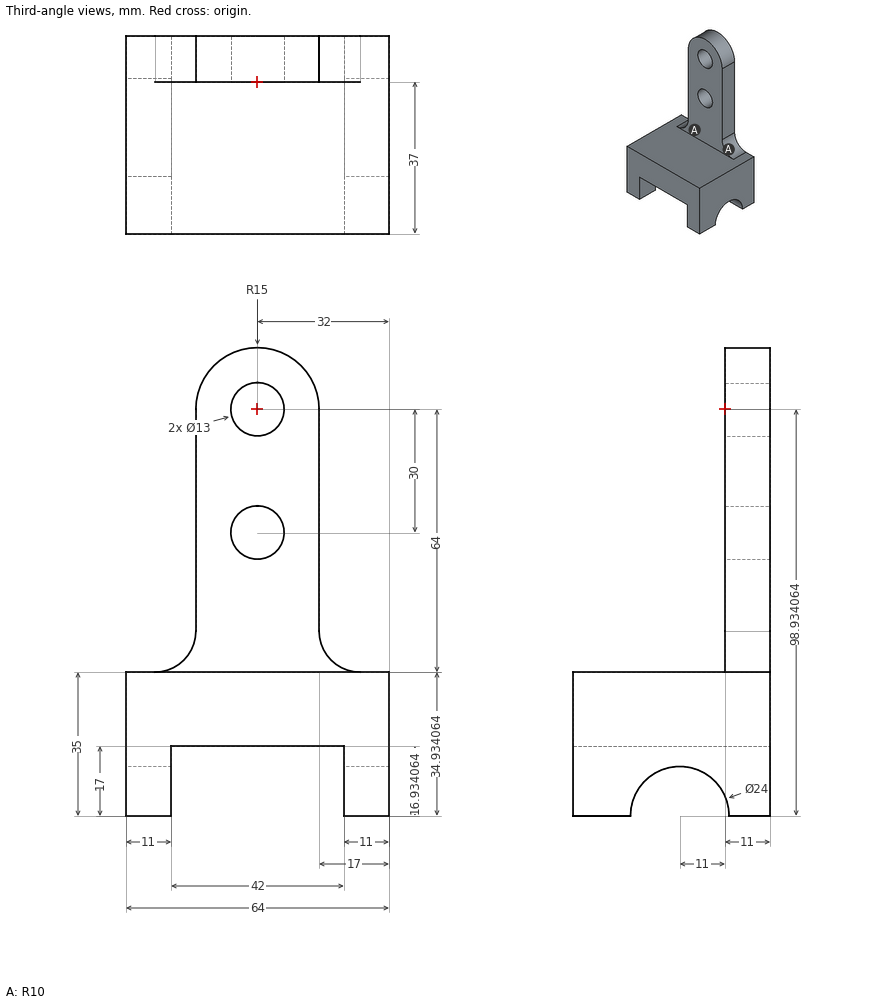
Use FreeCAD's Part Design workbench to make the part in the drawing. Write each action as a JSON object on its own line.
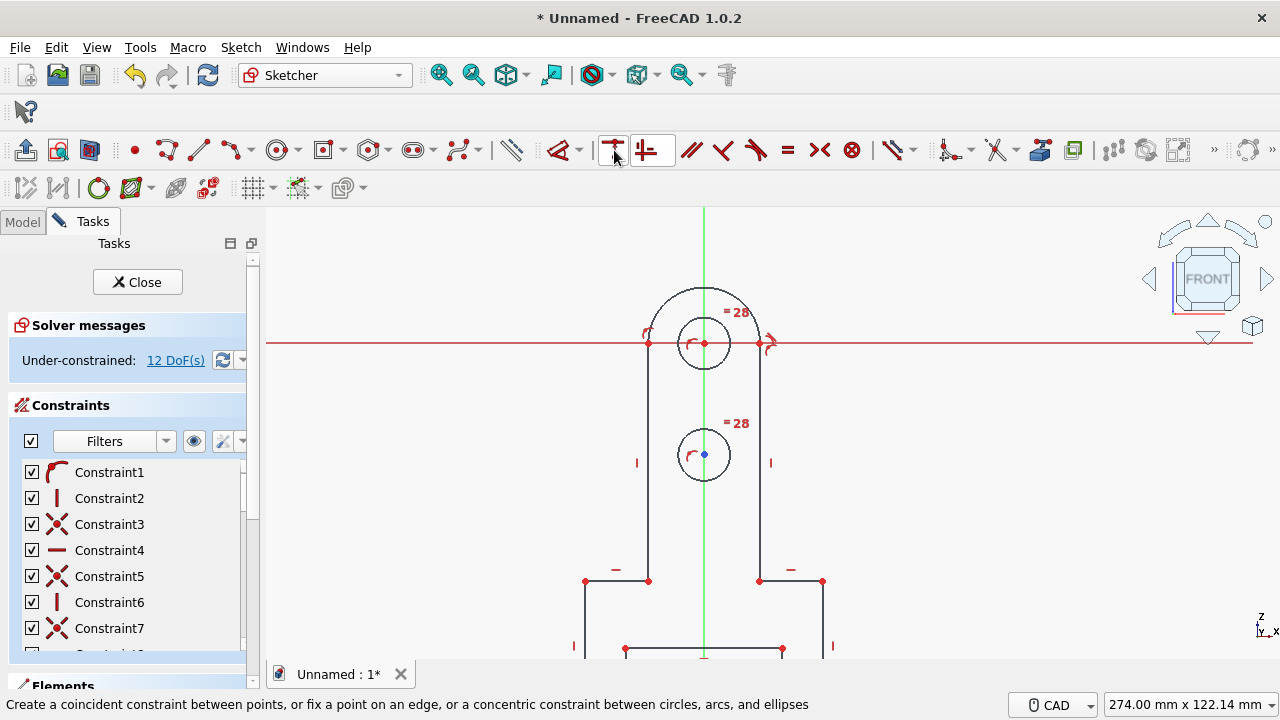
{"action": "left_click", "coordinate": [737, 298]}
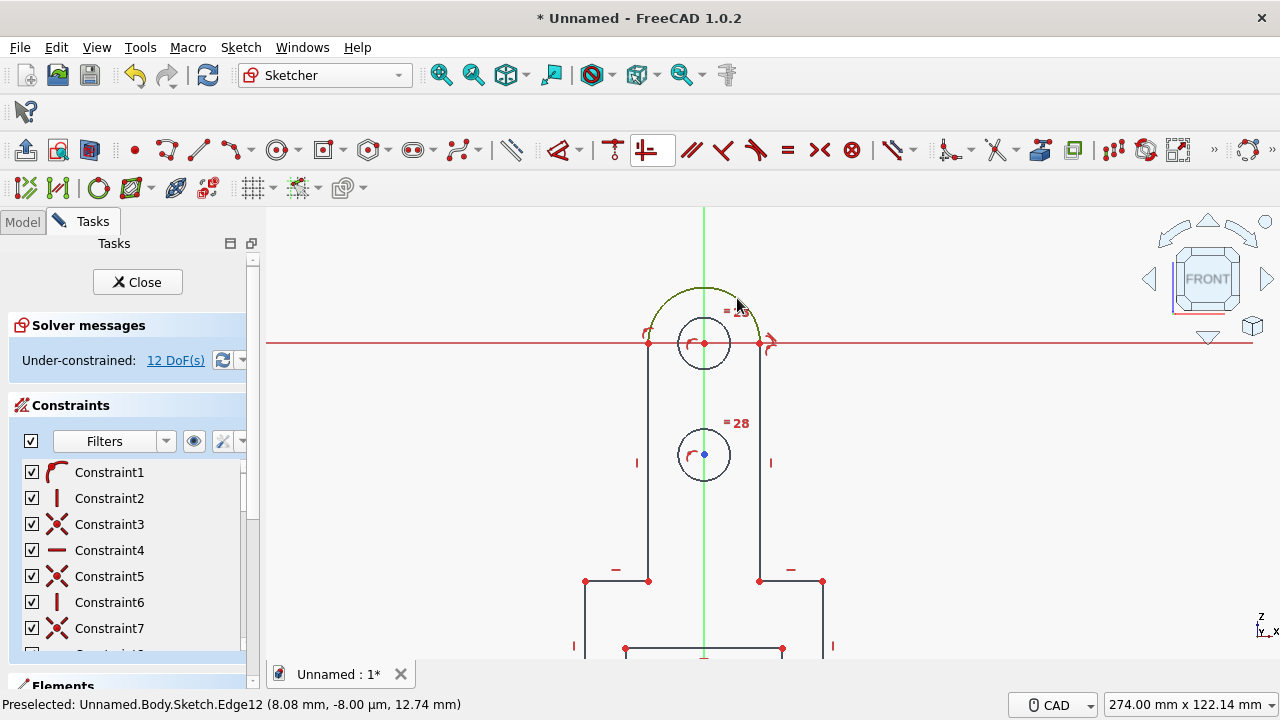
{"action": "left_click", "coordinate": [582, 150]}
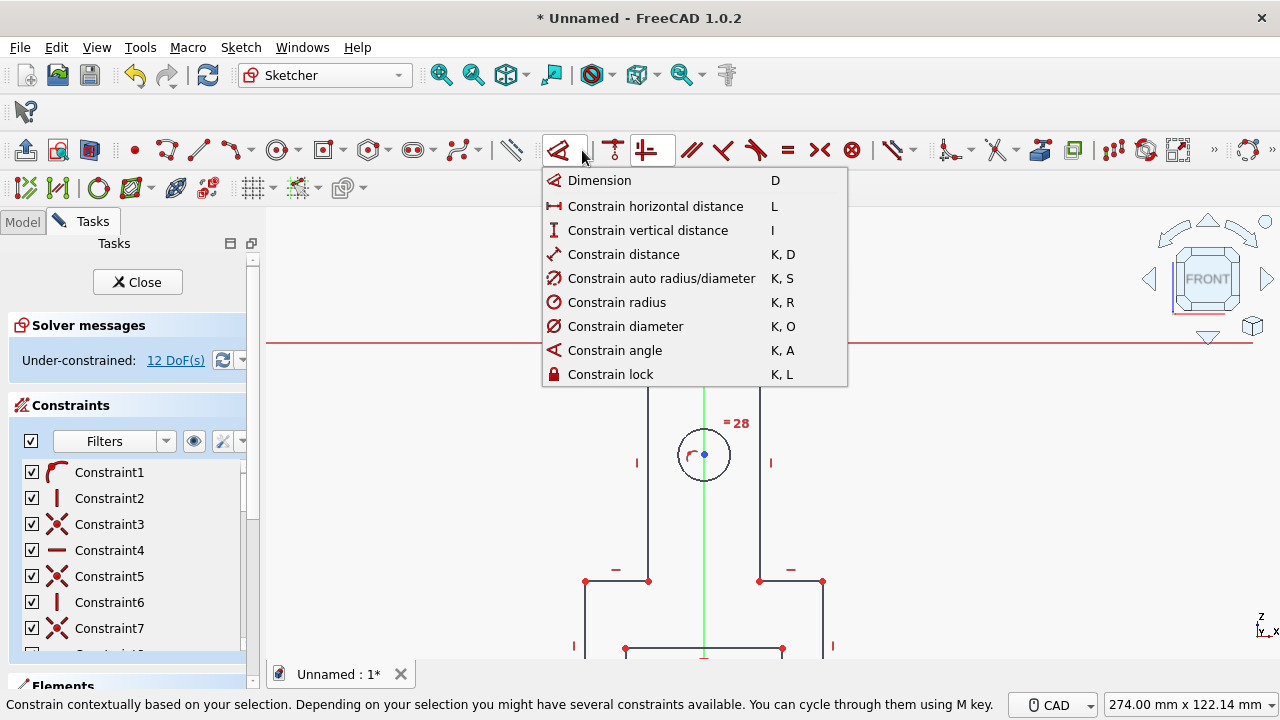
{"action": "left_click", "coordinate": [695, 302]}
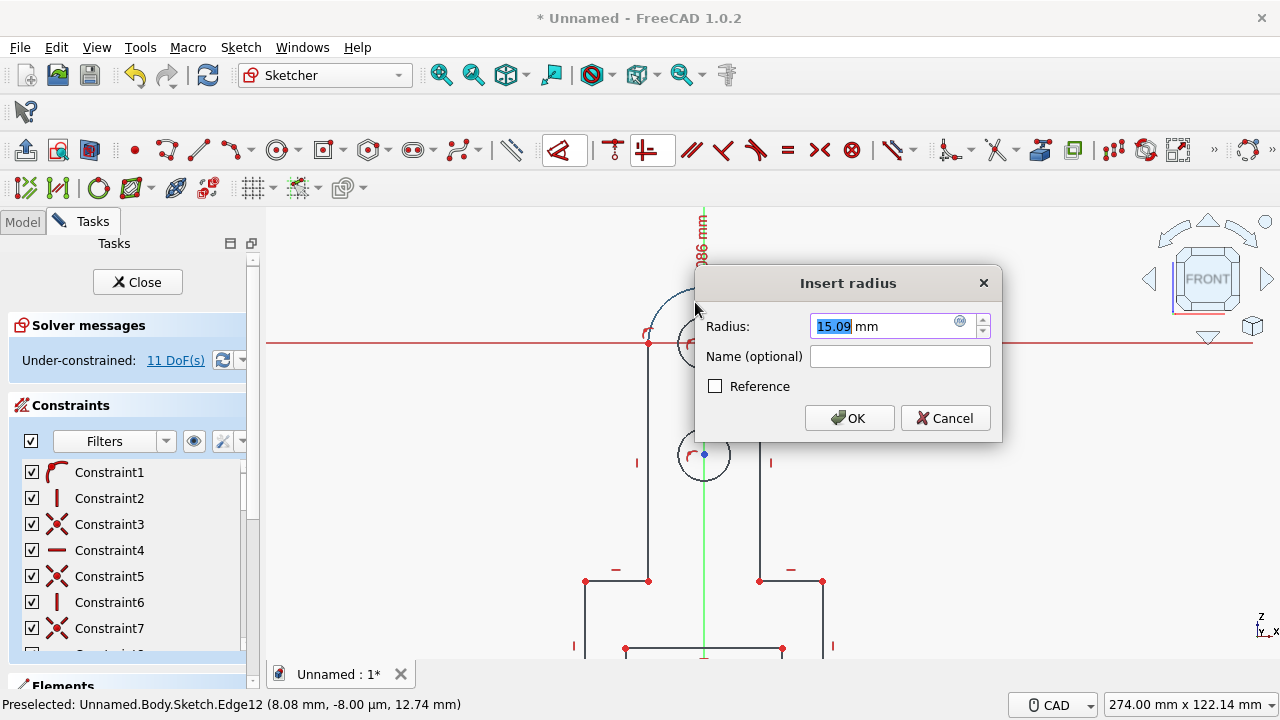
{"action": "type", "text": "15"}
{"action": "key", "text": "Return"}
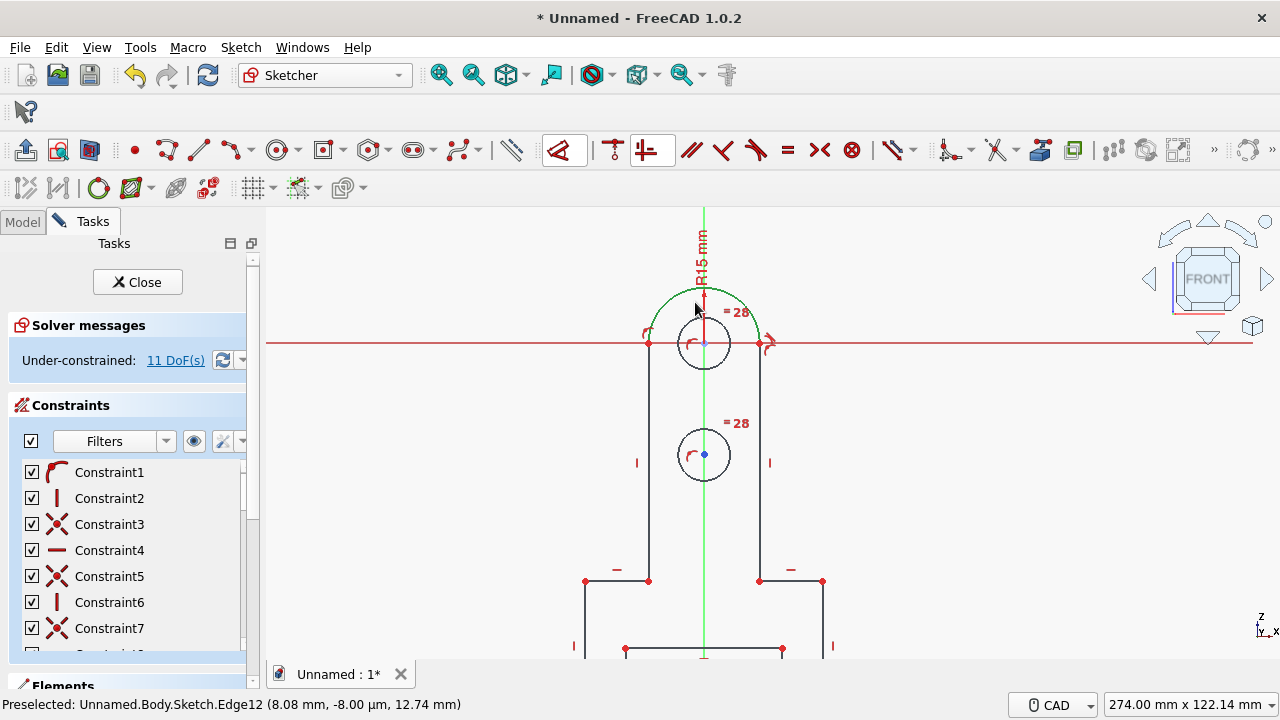
{"action": "left_click", "coordinate": [722, 325]}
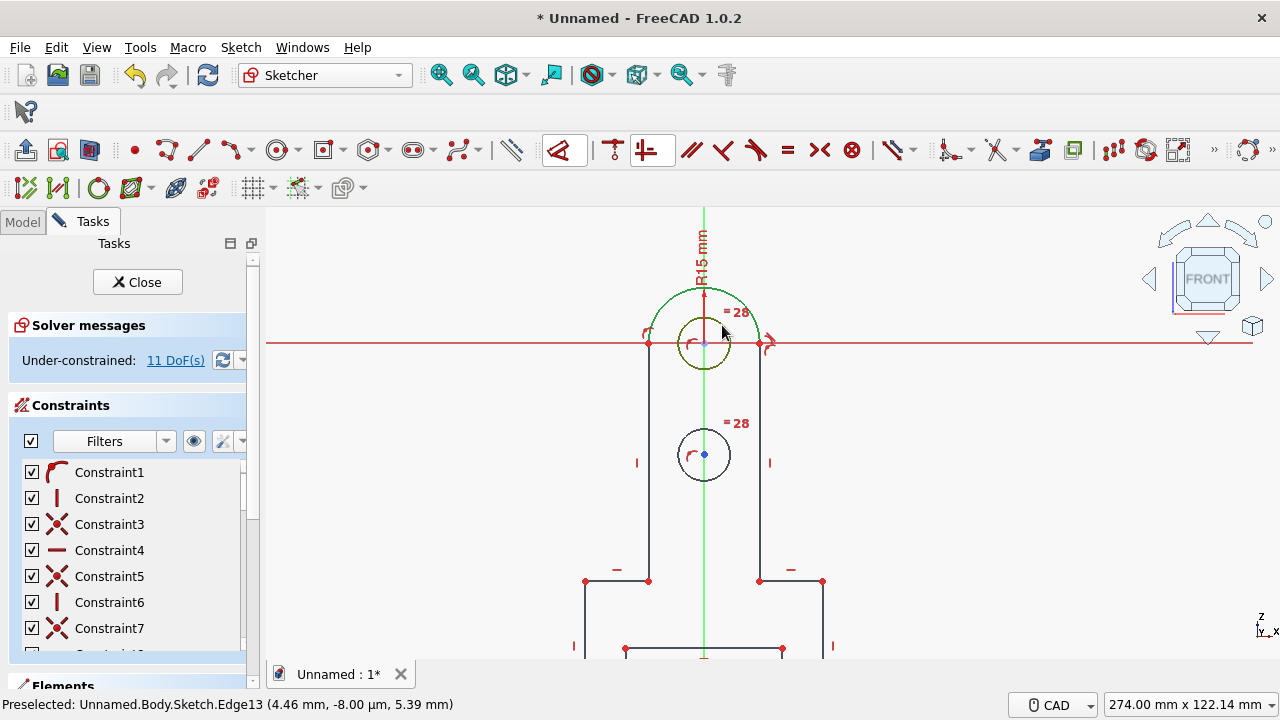
{"action": "left_click", "coordinate": [582, 150]}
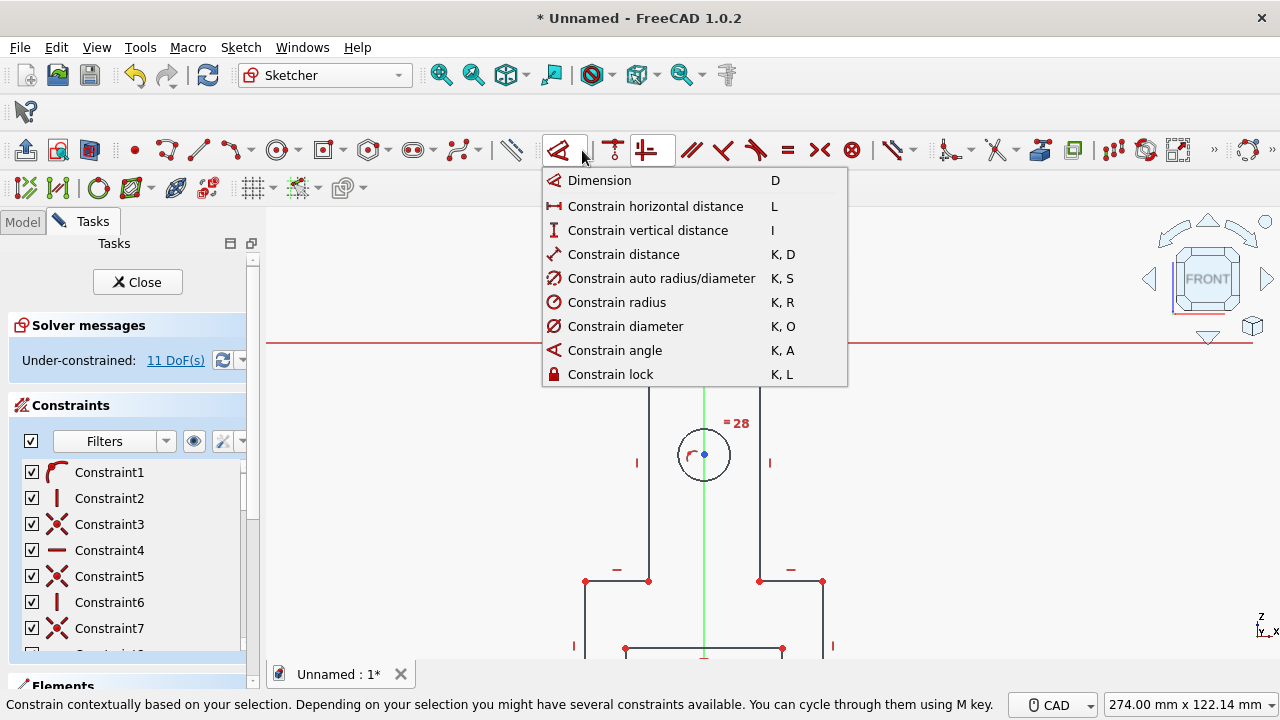
{"action": "left_click", "coordinate": [695, 326]}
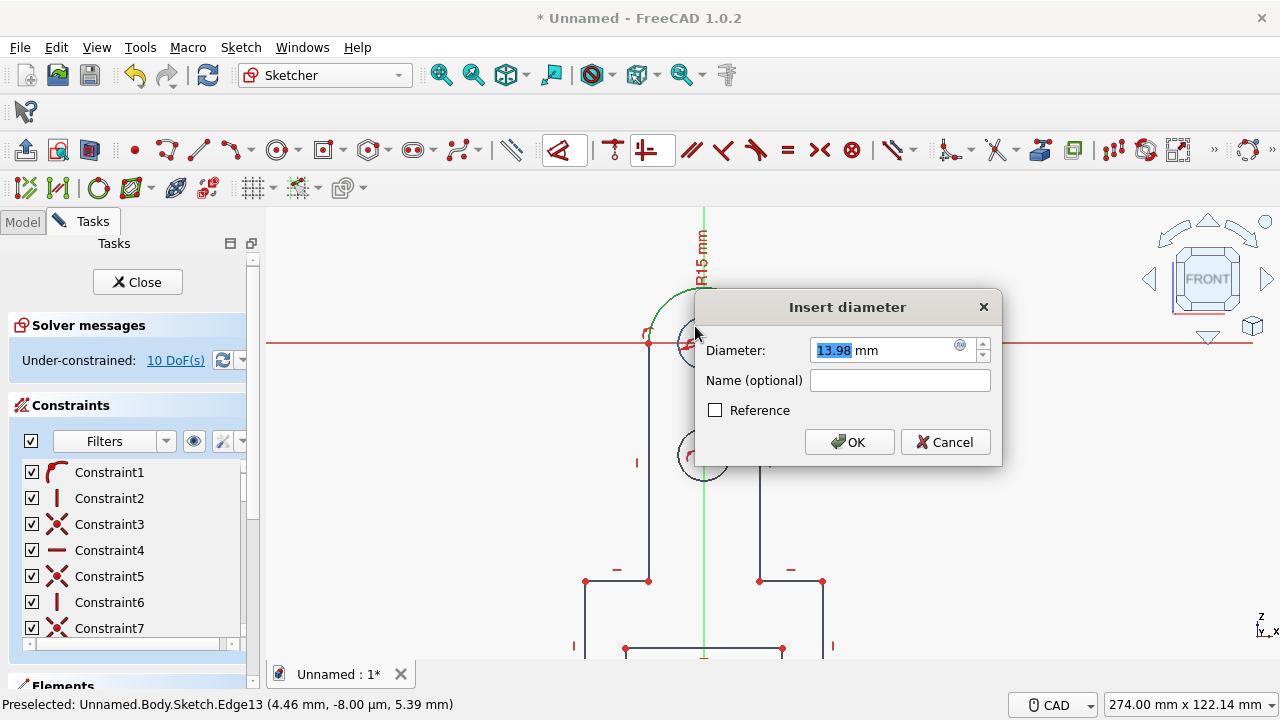
{"action": "type", "text": "13"}
{"action": "key", "text": "Return"}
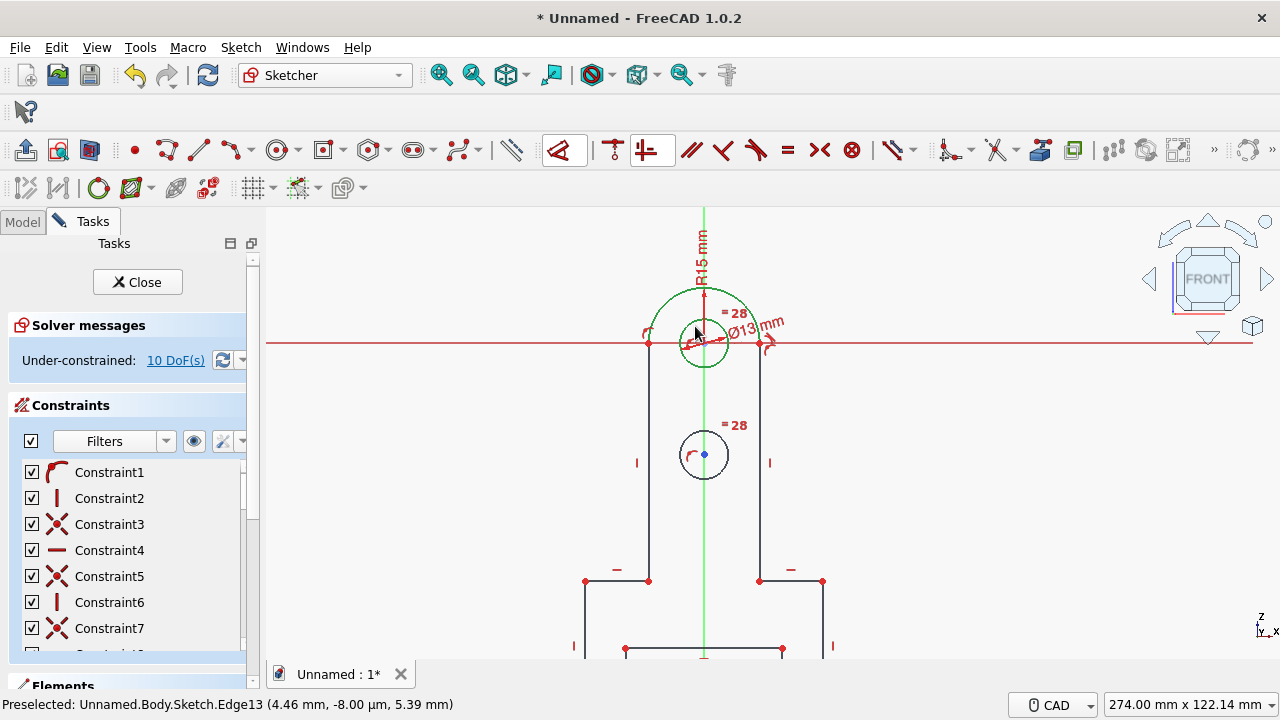
{"action": "left_click", "coordinate": [760, 415]}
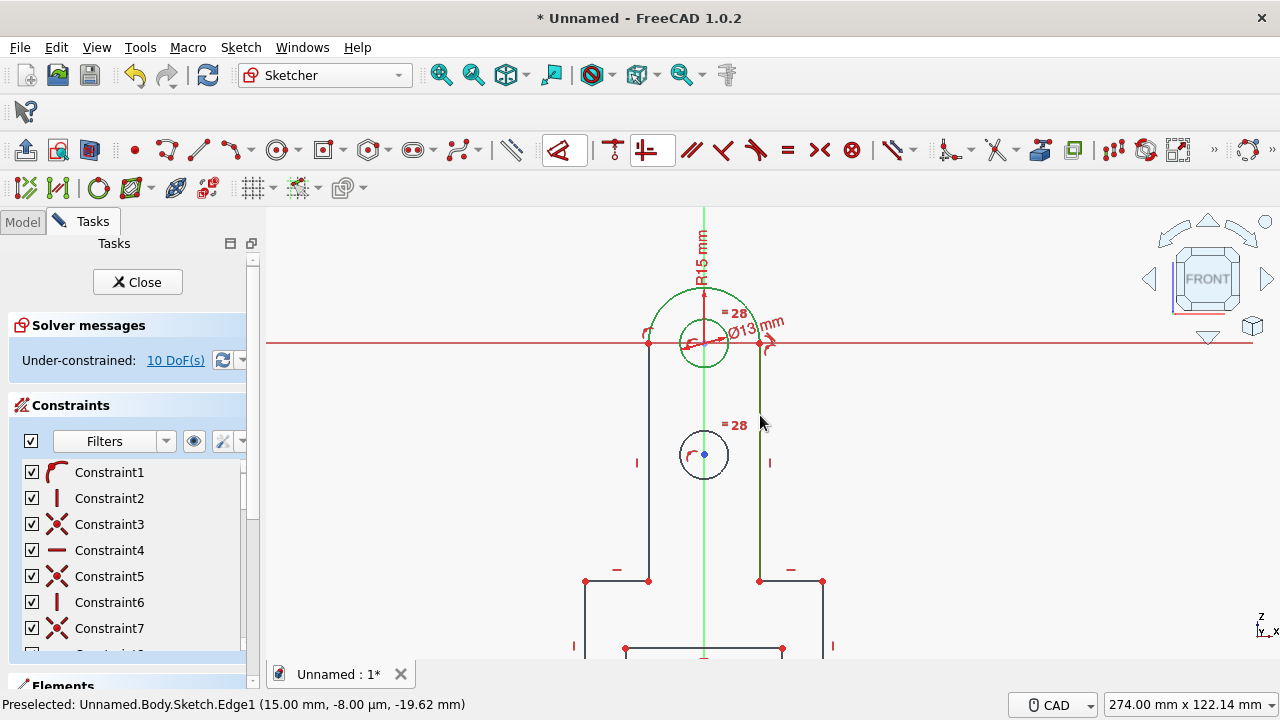
{"action": "left_click", "coordinate": [582, 150]}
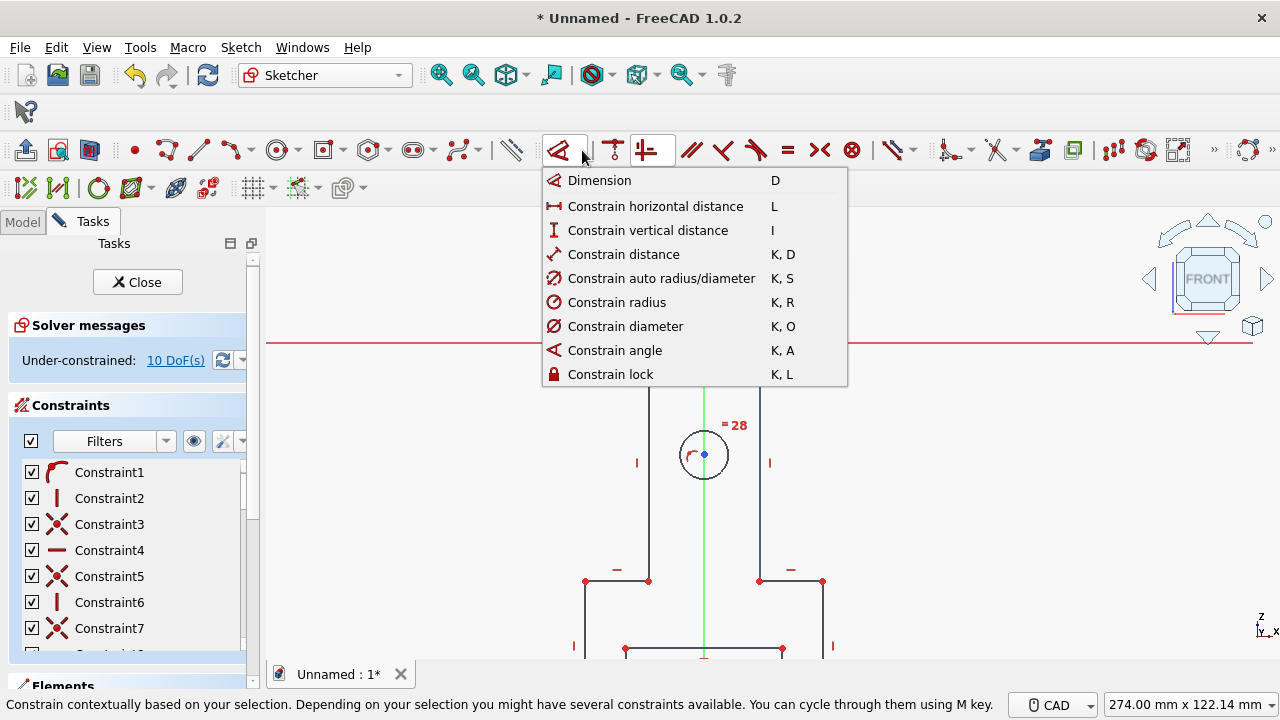
{"action": "left_click", "coordinate": [695, 230]}